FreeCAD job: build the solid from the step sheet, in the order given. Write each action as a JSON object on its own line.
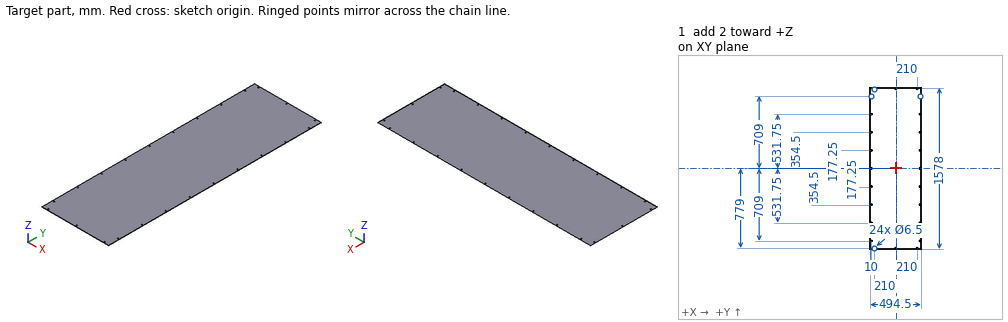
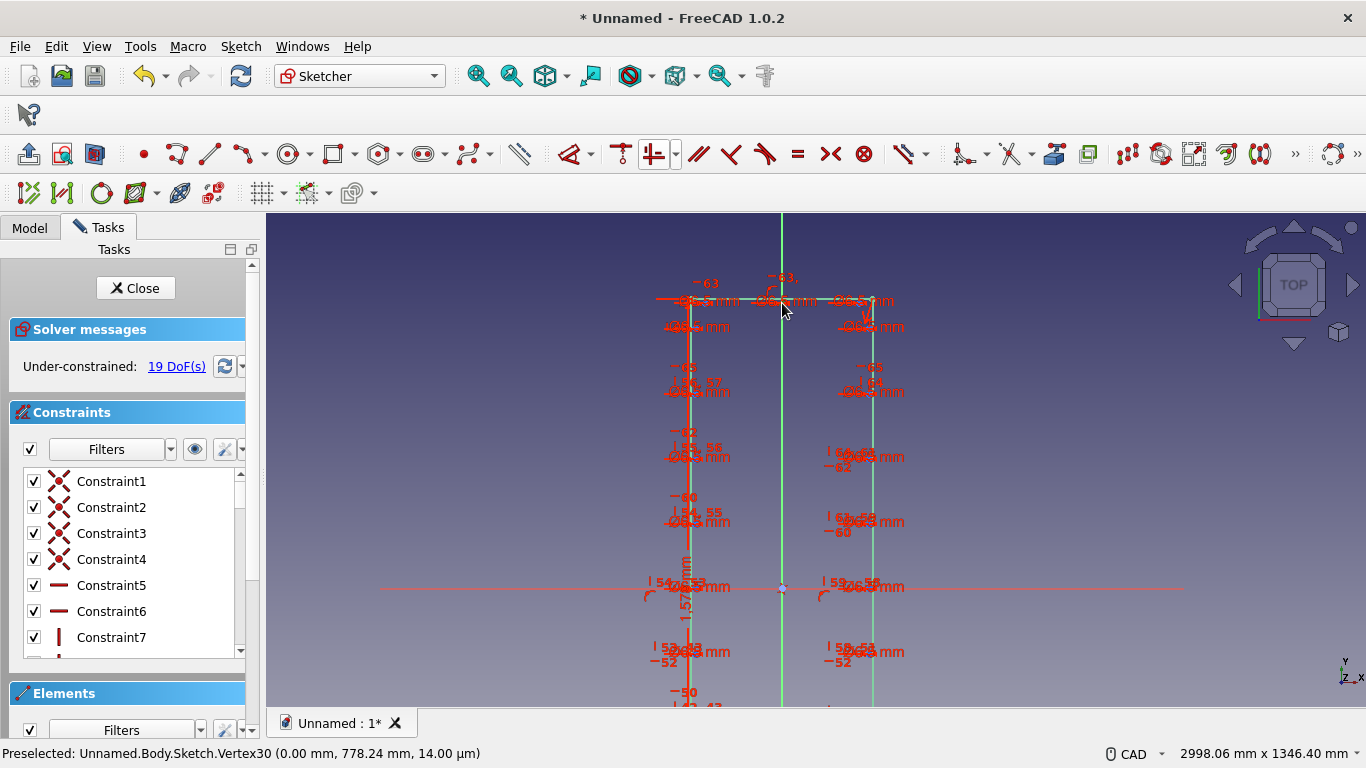
{"action": "left_click", "coordinate": [859, 303]}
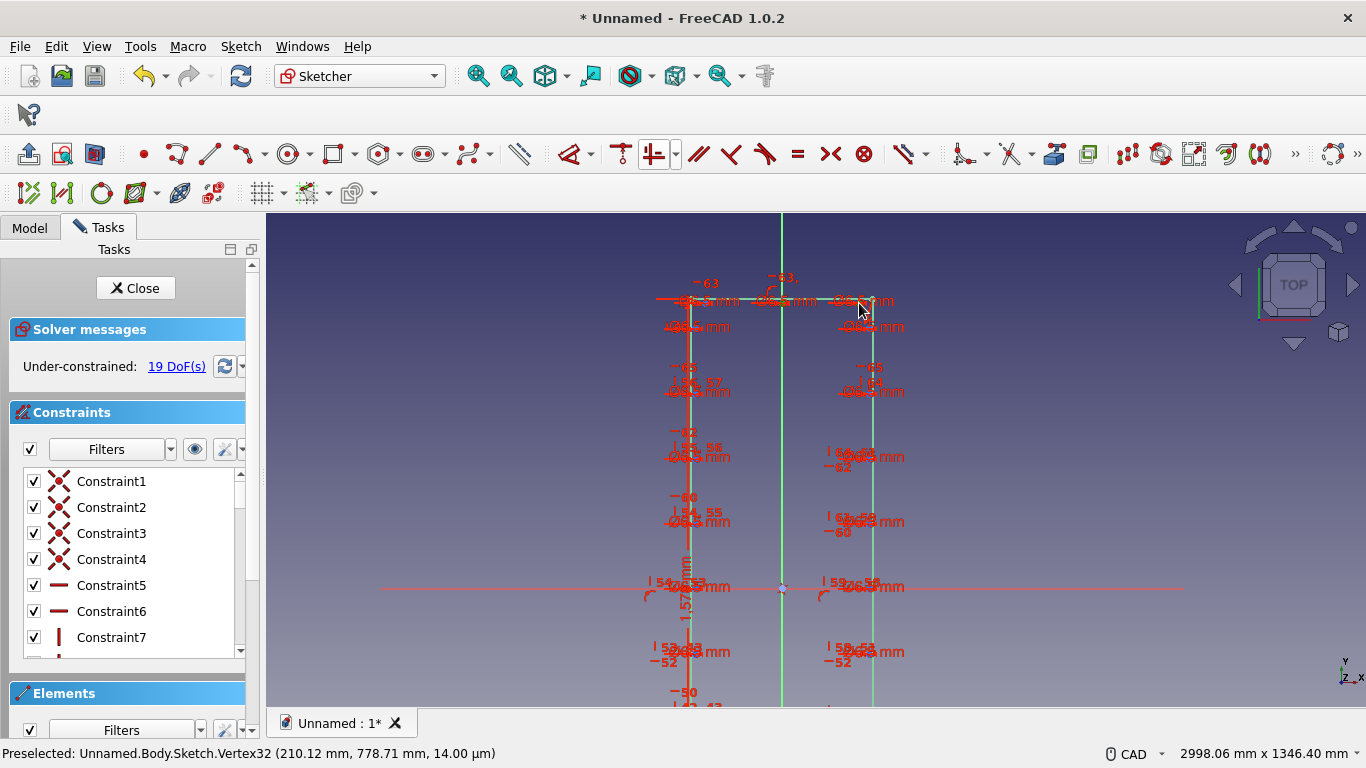
{"action": "key", "text": "h"}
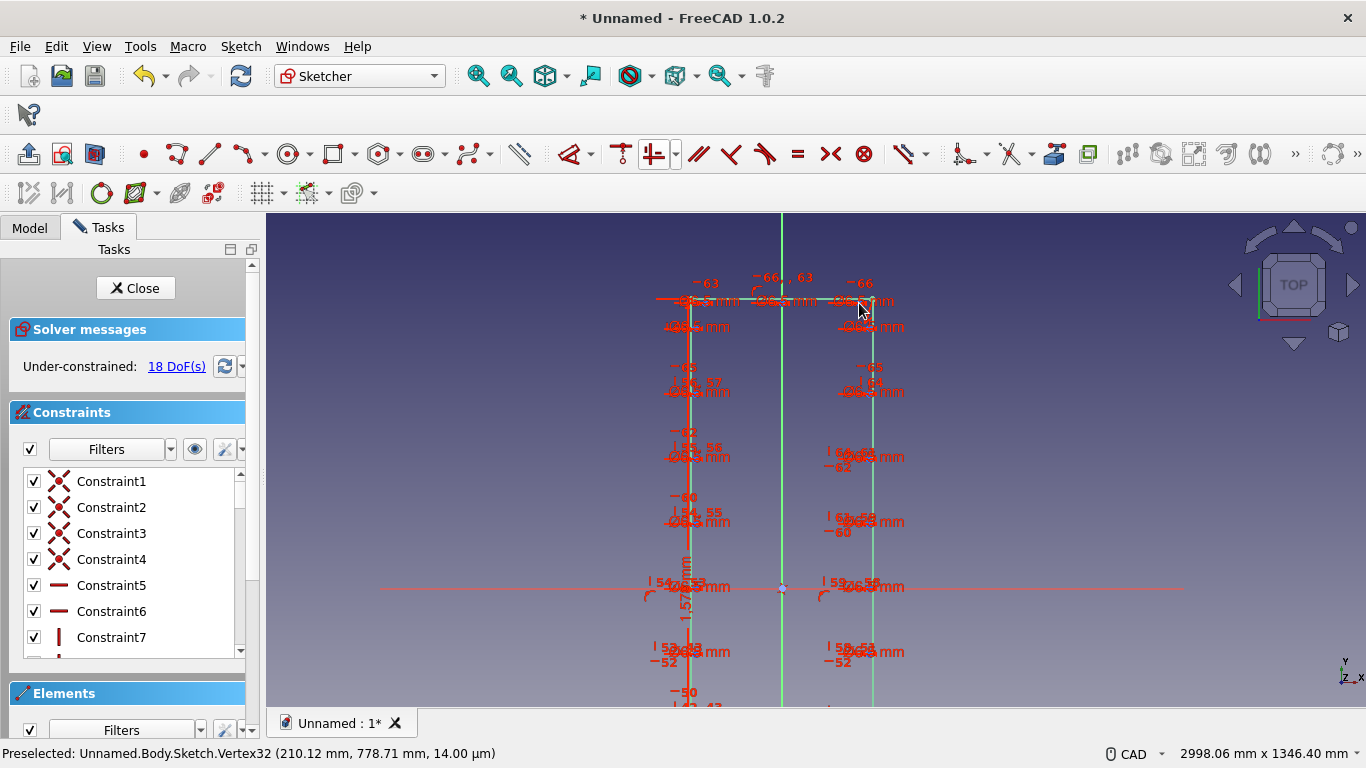
{"action": "left_click", "coordinate": [869, 394]}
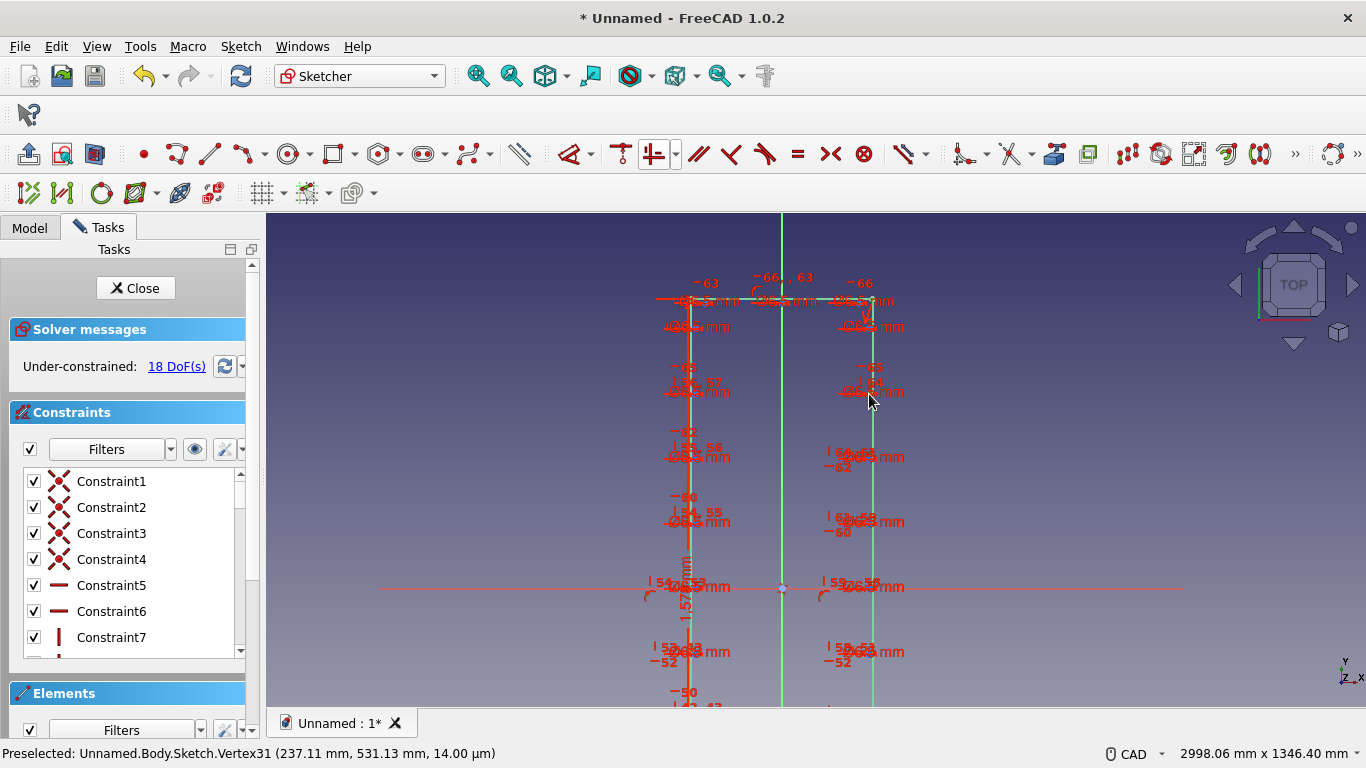
{"action": "left_click", "coordinate": [869, 329]}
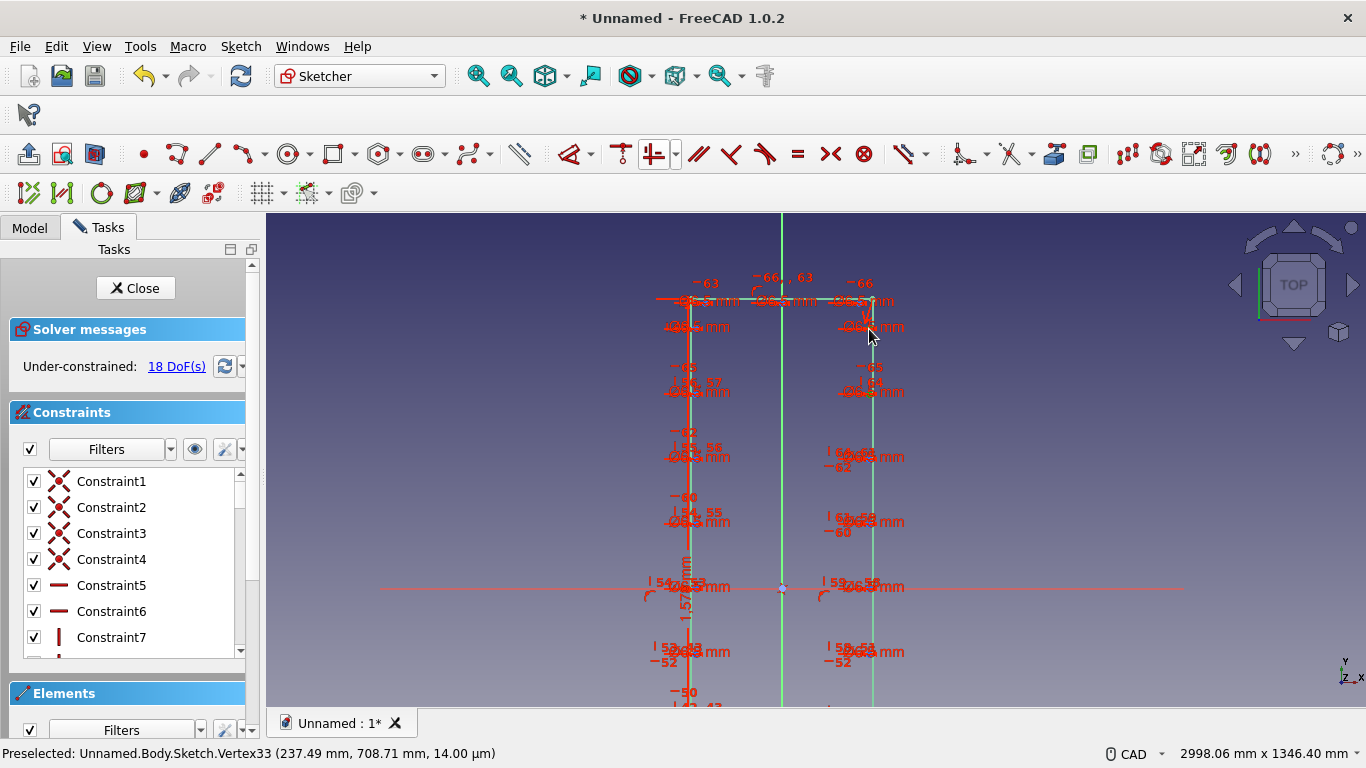
{"action": "key", "text": "v"}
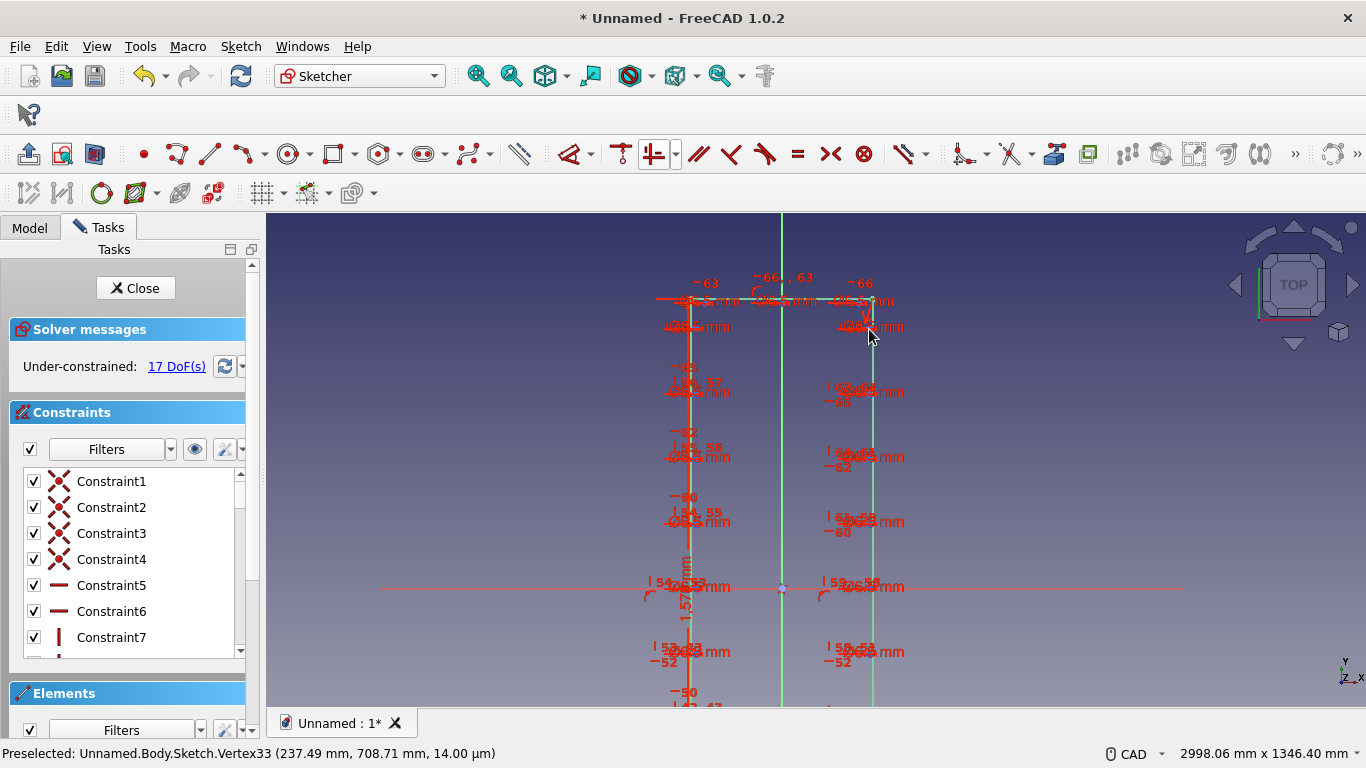
{"action": "scroll", "coordinate": [705, 303], "scroll_direction": "down", "scroll_amount": 3}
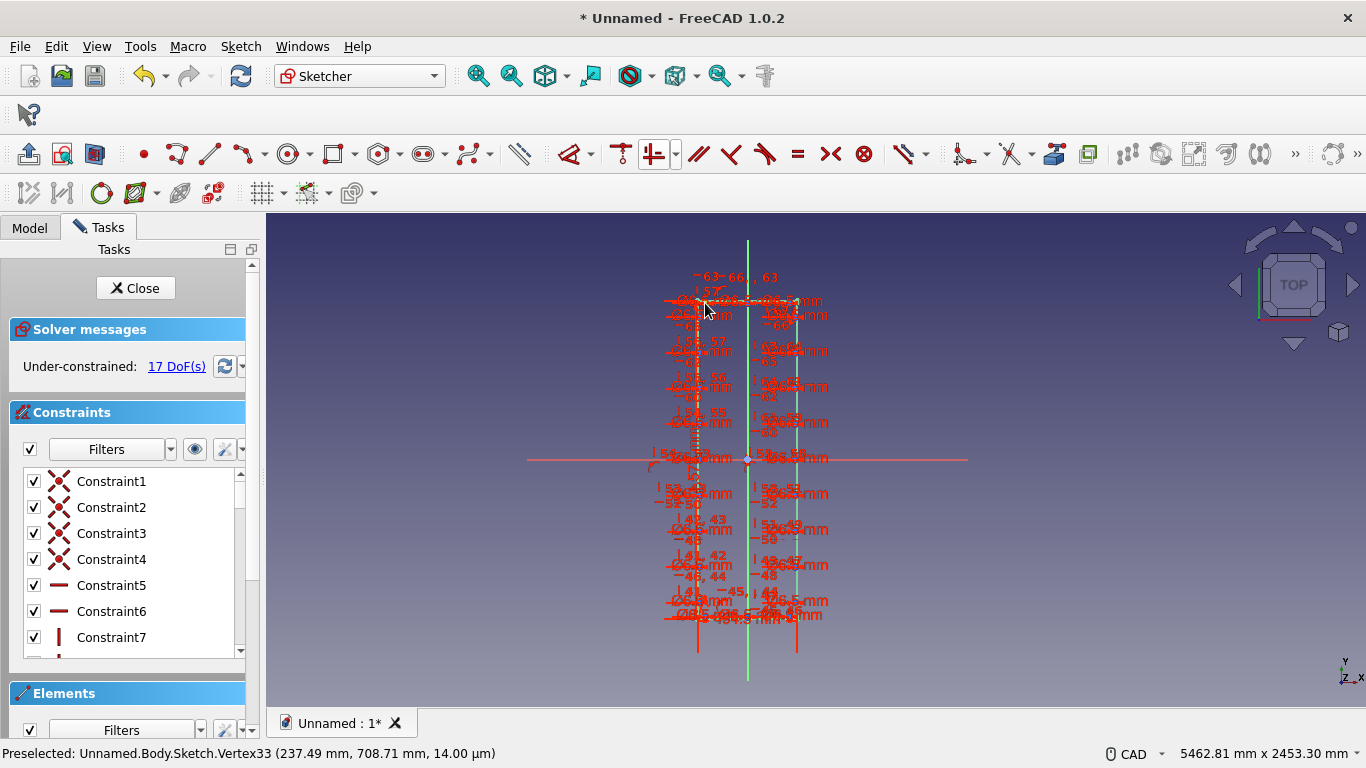
{"action": "scroll", "coordinate": [705, 617], "scroll_direction": "up", "scroll_amount": 3}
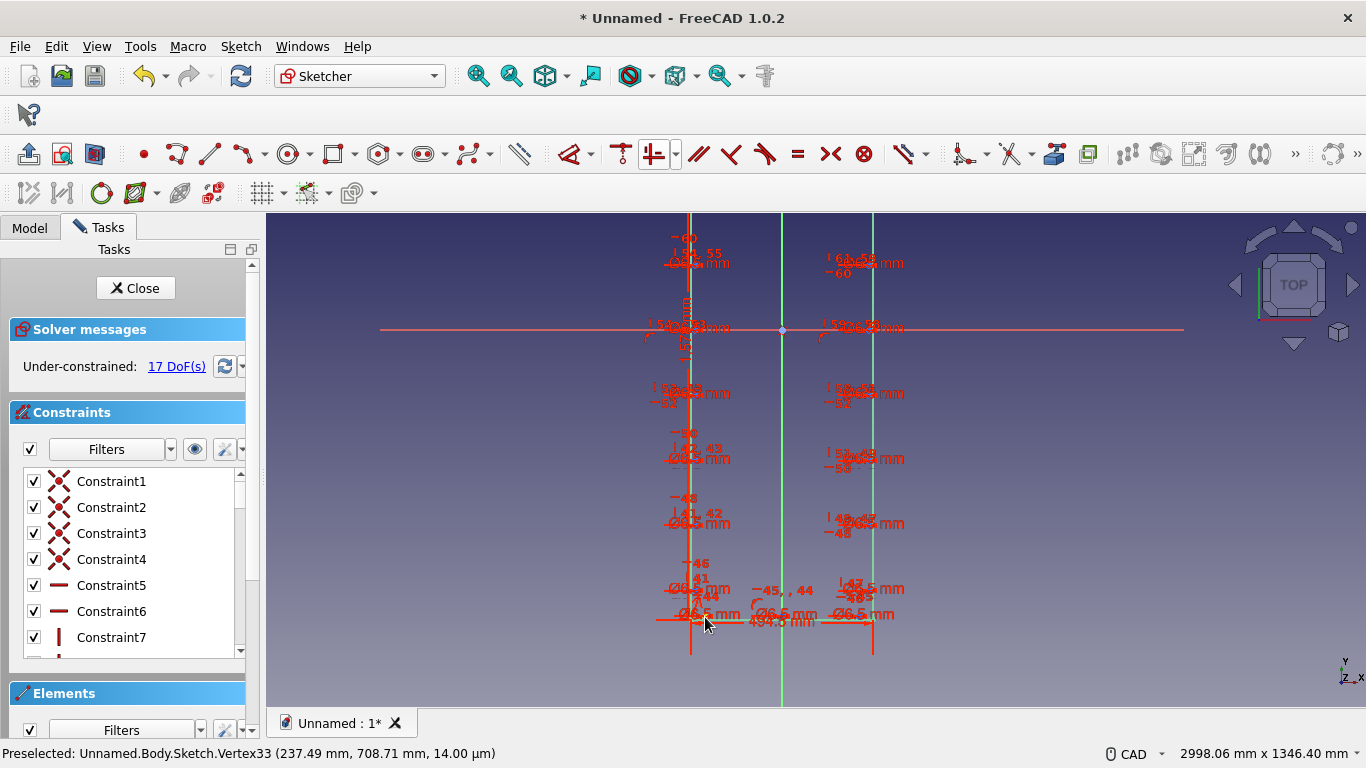
{"action": "left_click", "coordinate": [705, 616]}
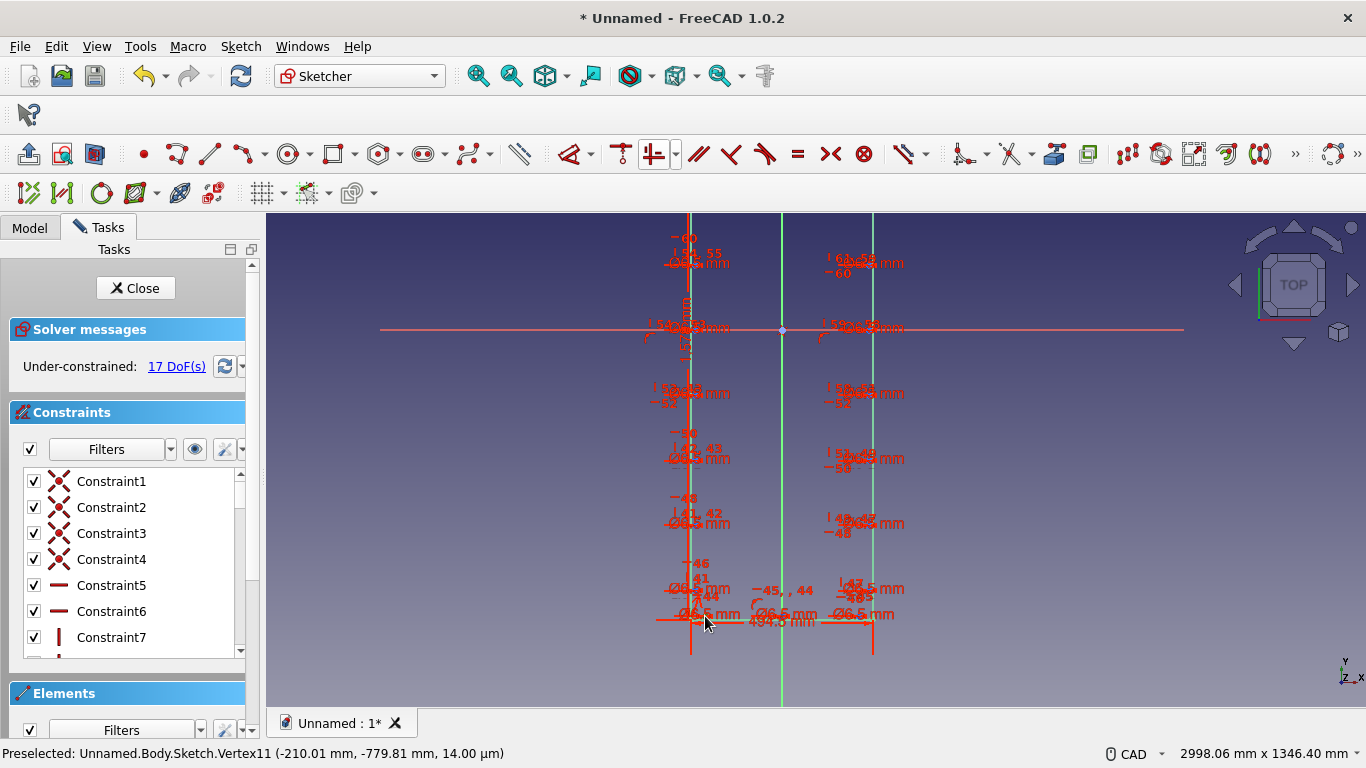
{"action": "scroll", "coordinate": [705, 618], "scroll_direction": "down", "scroll_amount": 3}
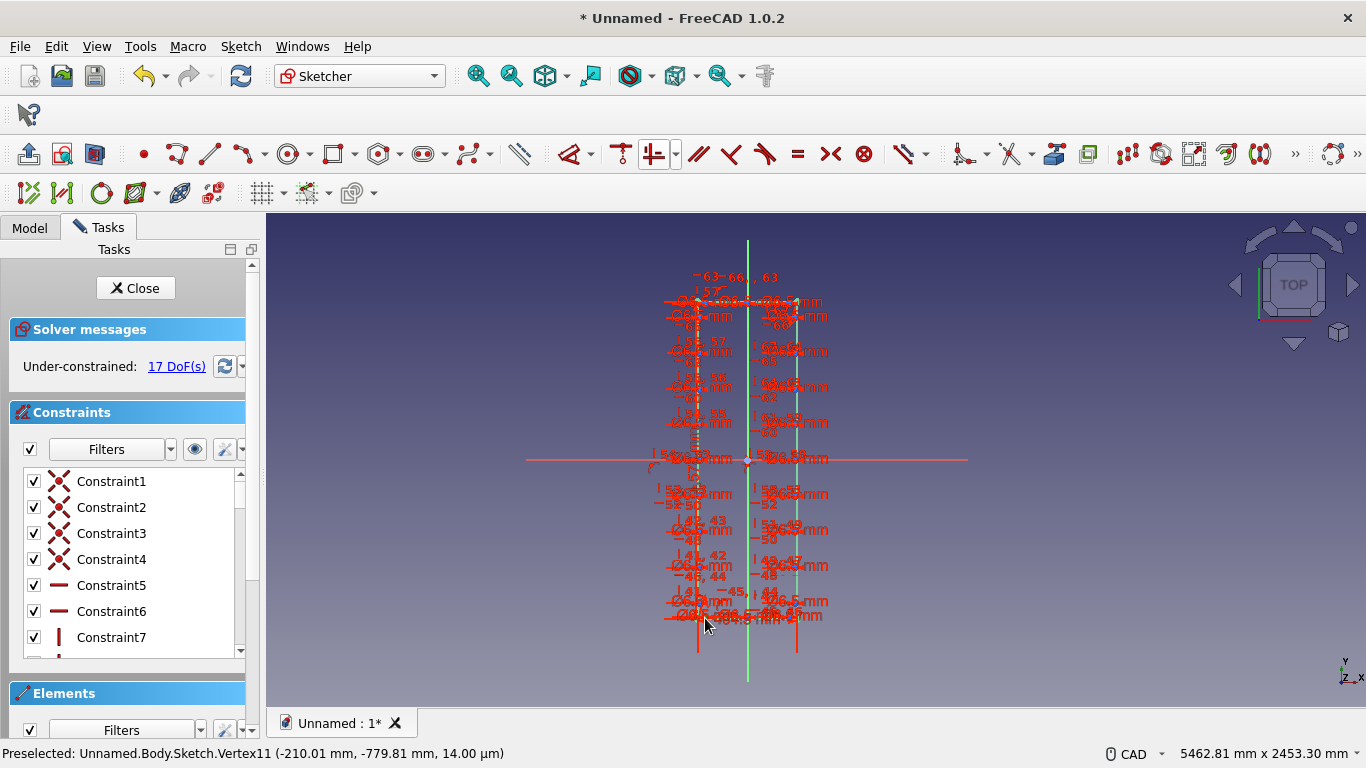
{"action": "scroll", "coordinate": [705, 304], "scroll_direction": "up", "scroll_amount": 3}